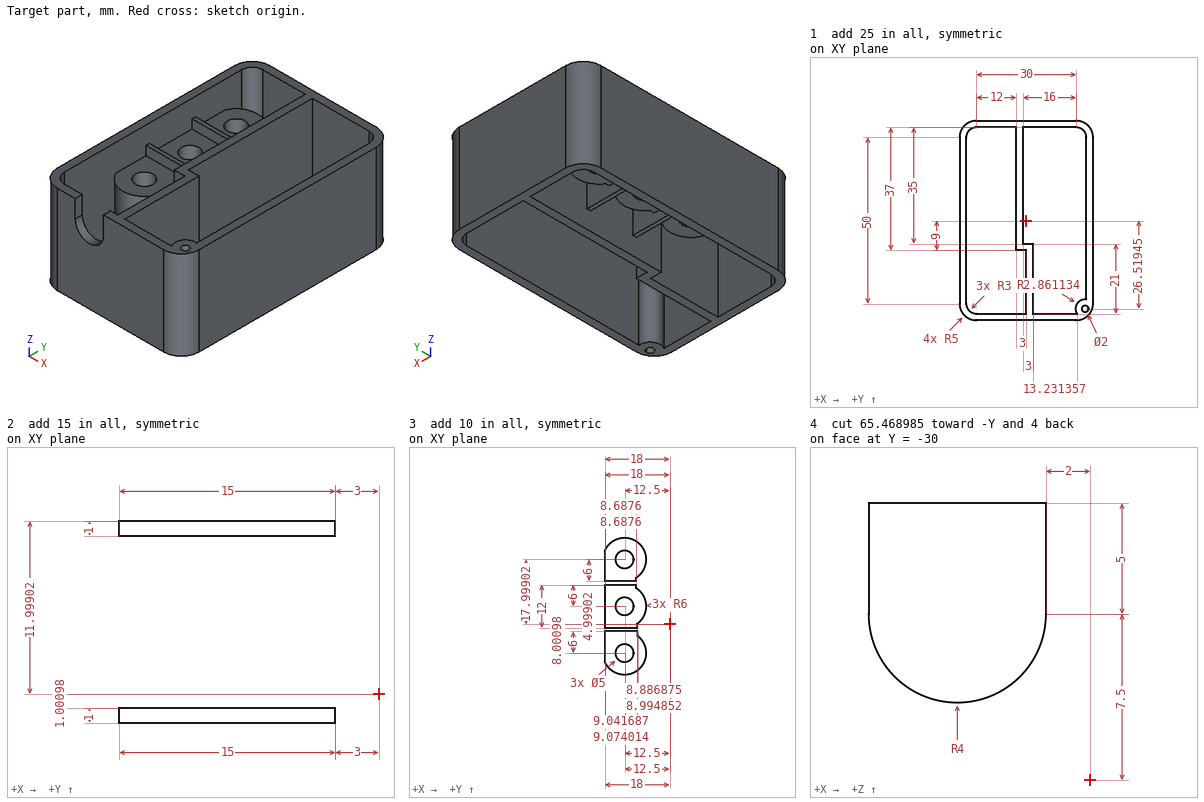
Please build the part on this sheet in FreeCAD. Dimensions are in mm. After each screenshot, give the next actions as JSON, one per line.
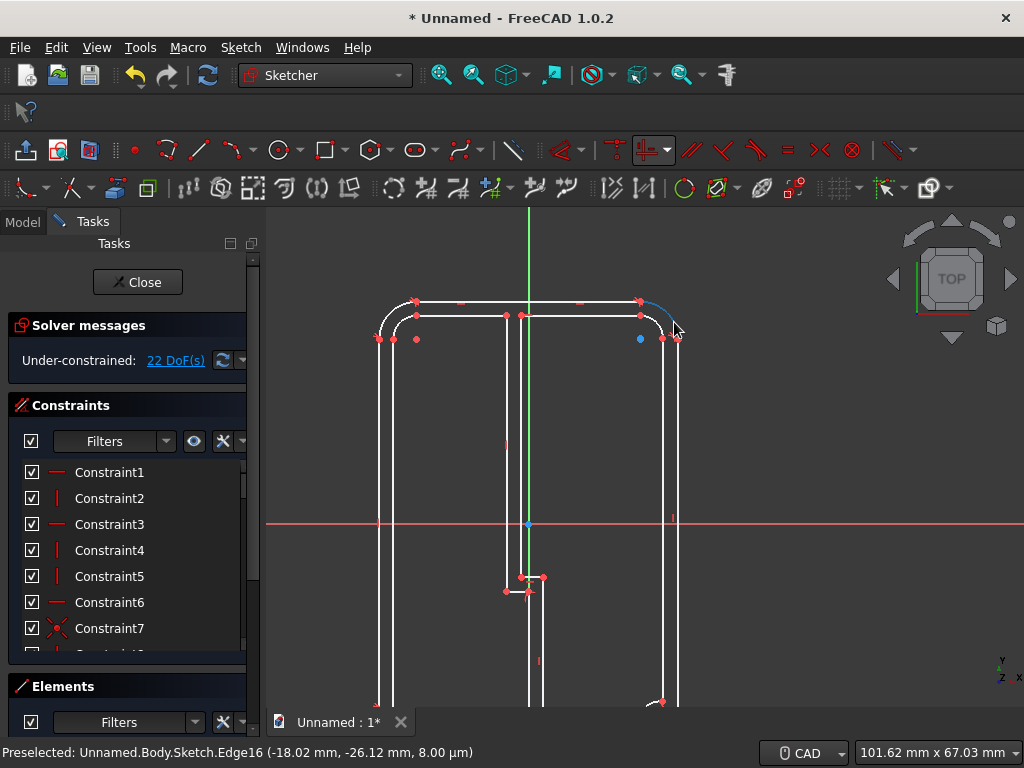
{"action": "left_click", "coordinate": [674, 322]}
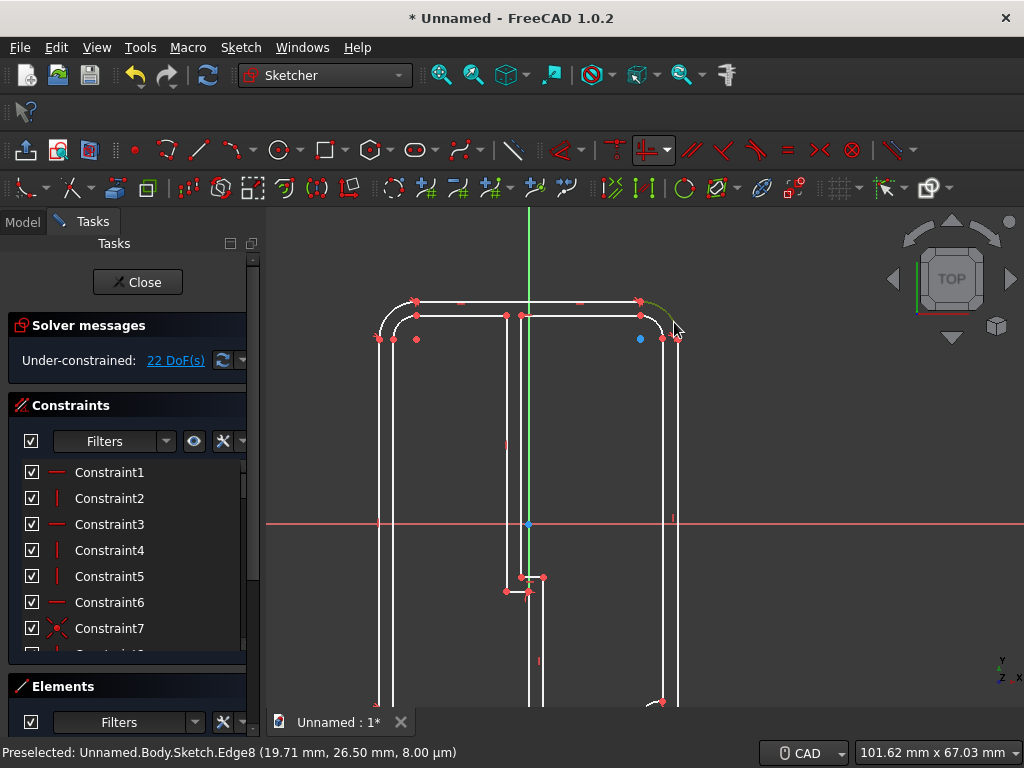
{"action": "scroll", "coordinate": [660, 328], "scroll_direction": "up", "scroll_amount": 2}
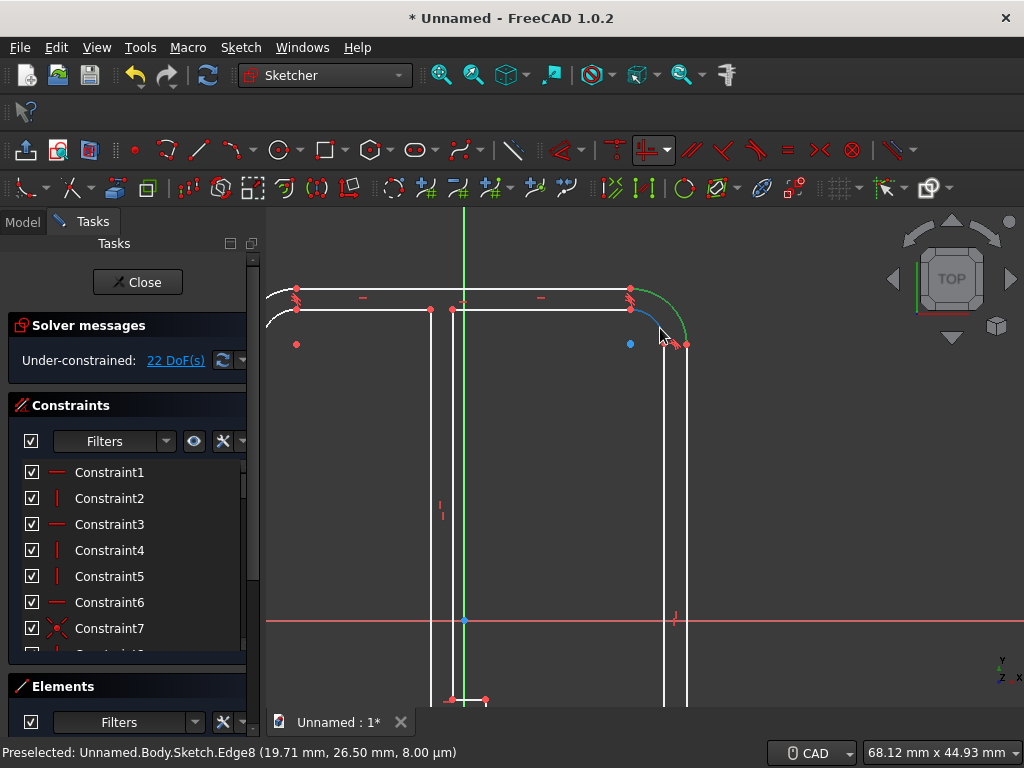
{"action": "left_click", "coordinate": [660, 328]}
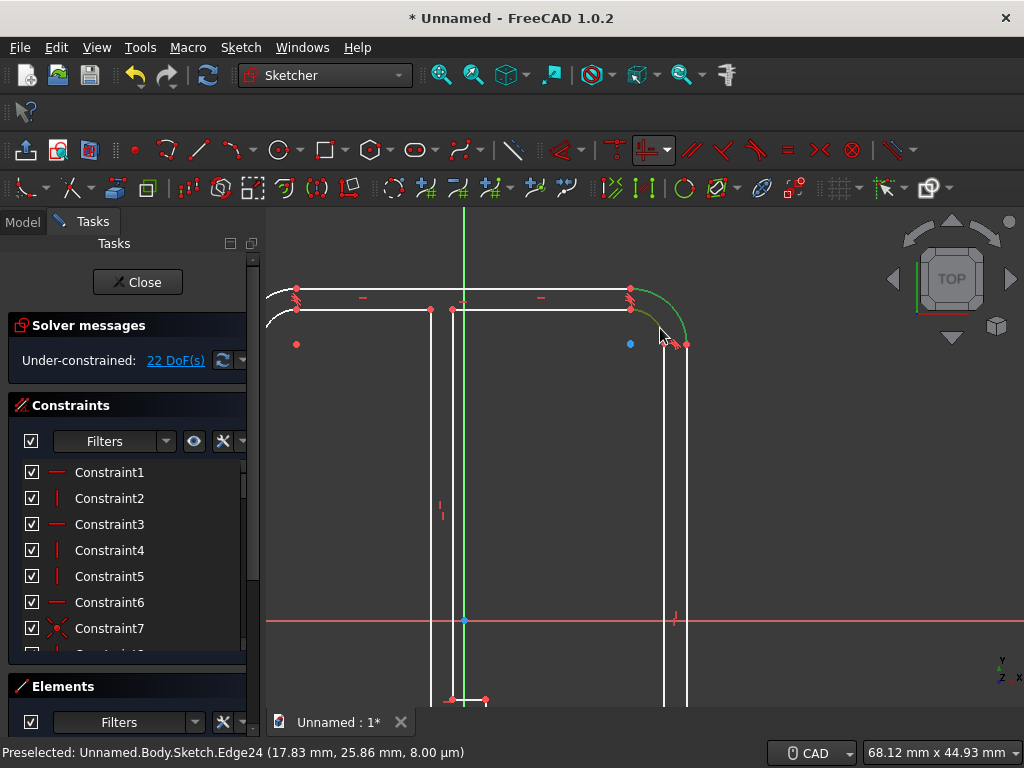
{"action": "left_click", "coordinate": [616, 150]}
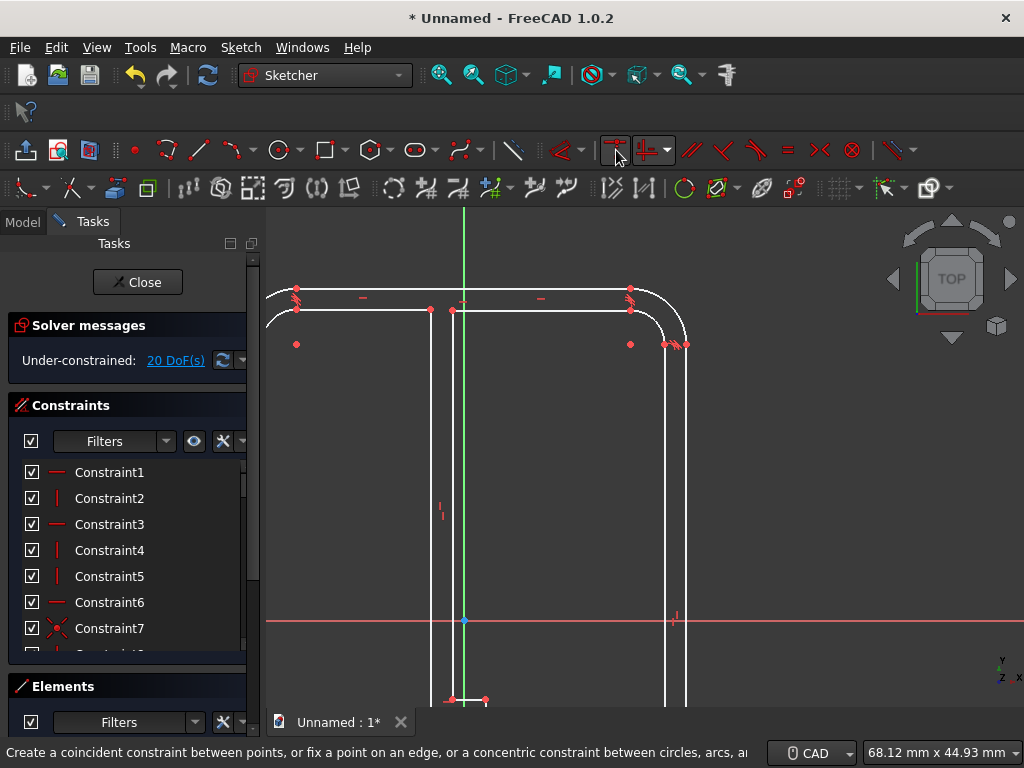
{"action": "scroll", "coordinate": [668, 324], "scroll_direction": "down", "scroll_amount": 4}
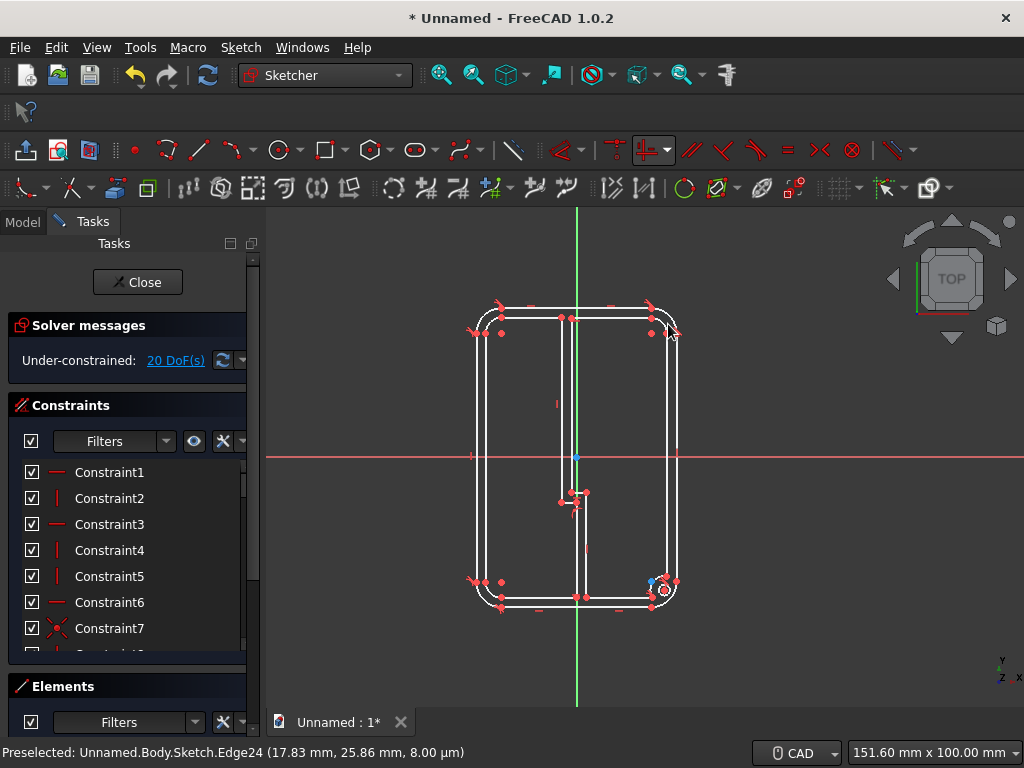
{"action": "scroll", "coordinate": [490, 311], "scroll_direction": "up", "scroll_amount": 2}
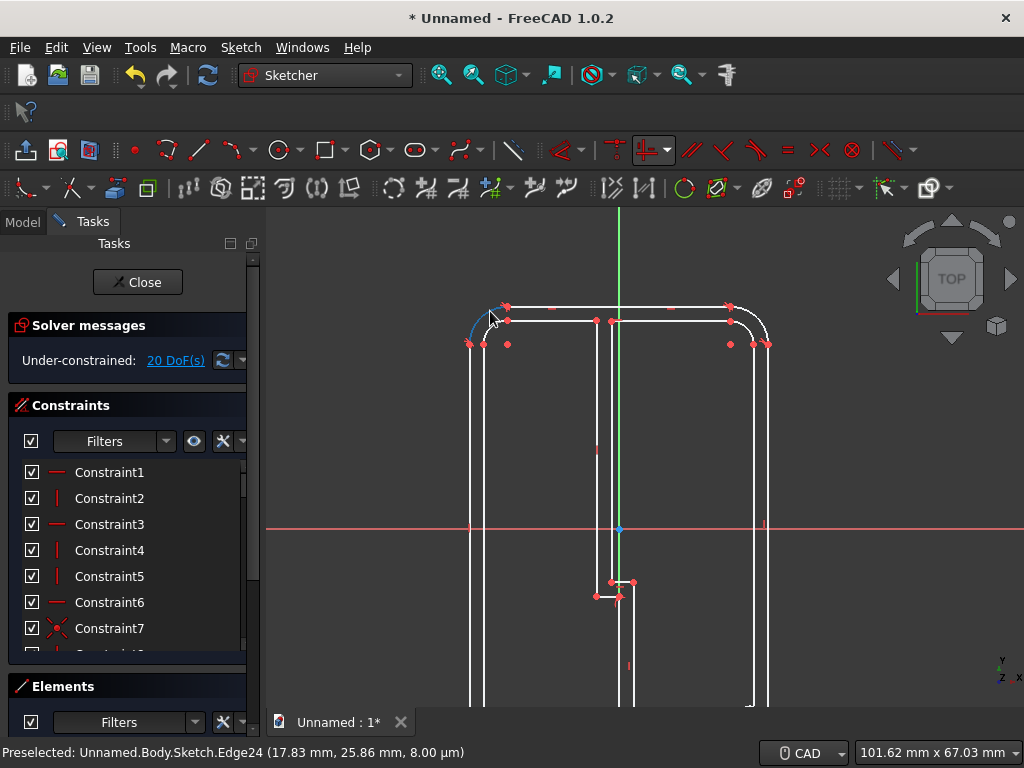
{"action": "left_click", "coordinate": [490, 311]}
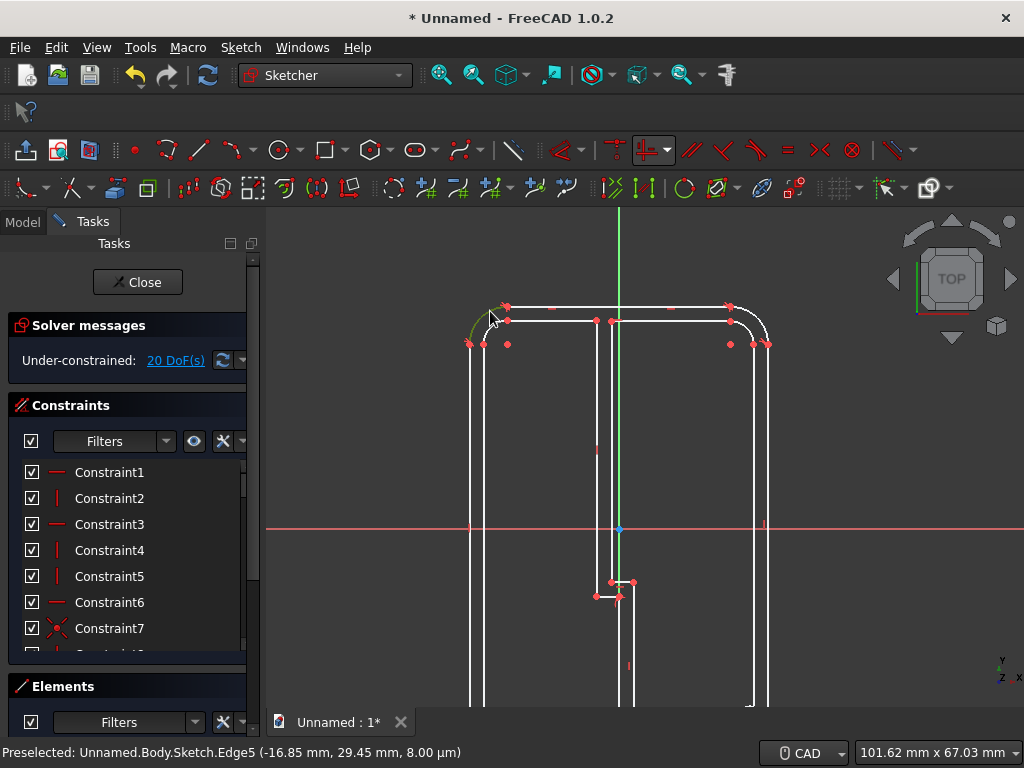
{"action": "scroll", "coordinate": [490, 310], "scroll_direction": "down", "scroll_amount": 2}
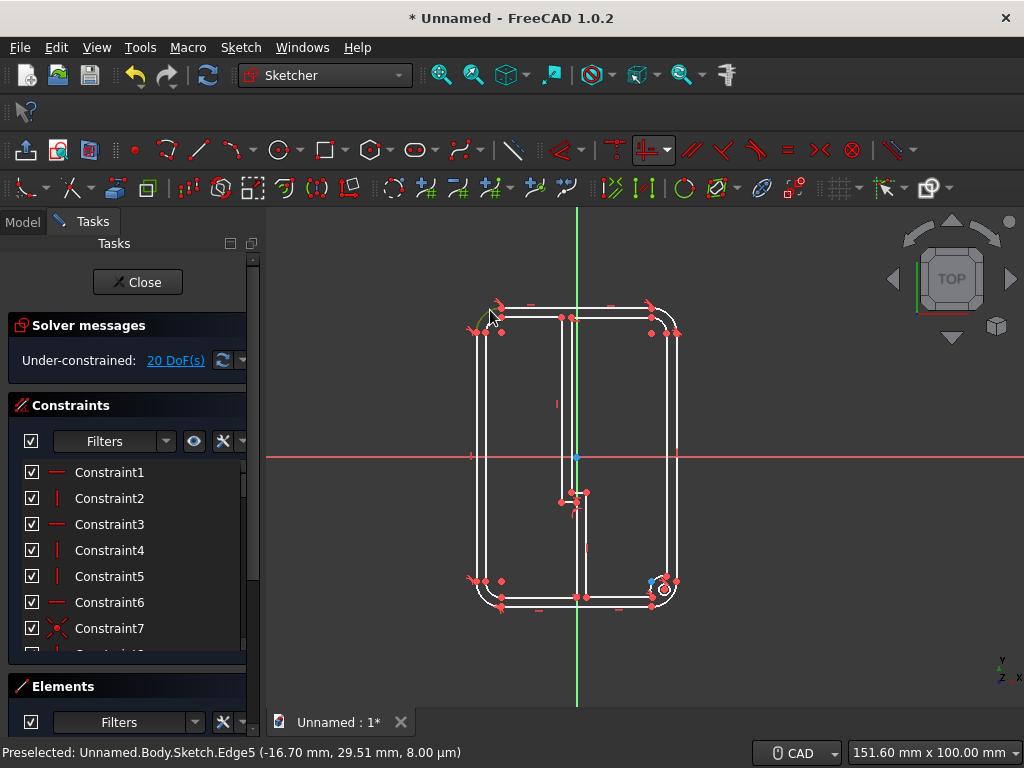
{"action": "scroll", "coordinate": [479, 593], "scroll_direction": "up", "scroll_amount": 2}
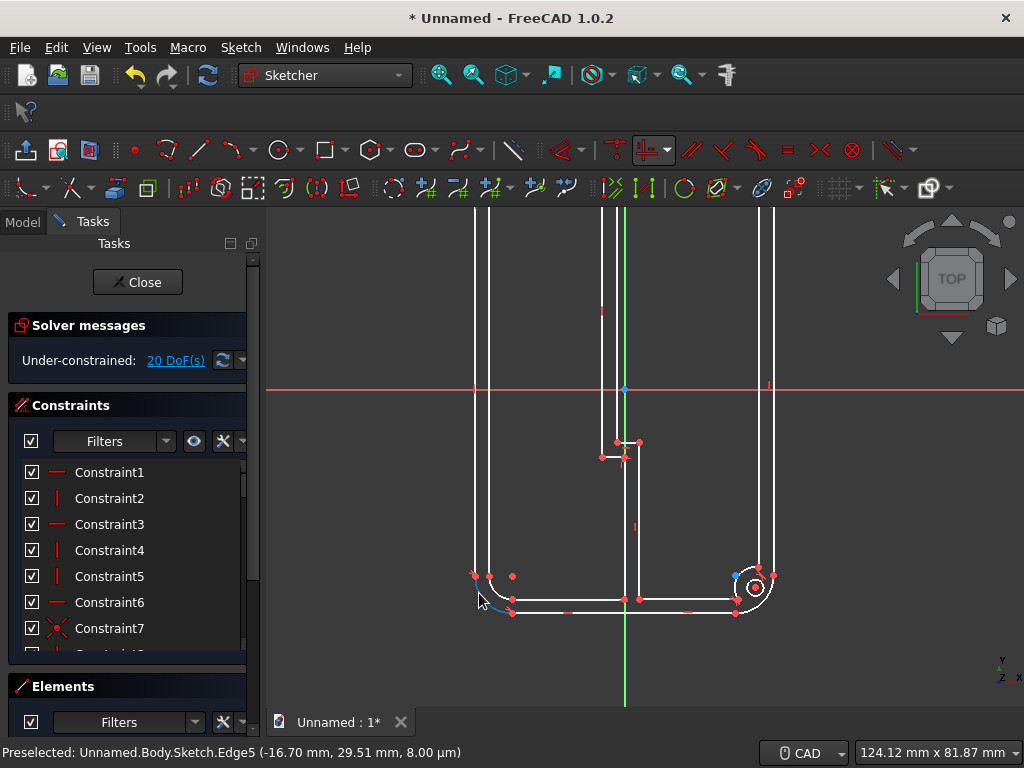
{"action": "left_click", "coordinate": [479, 593]}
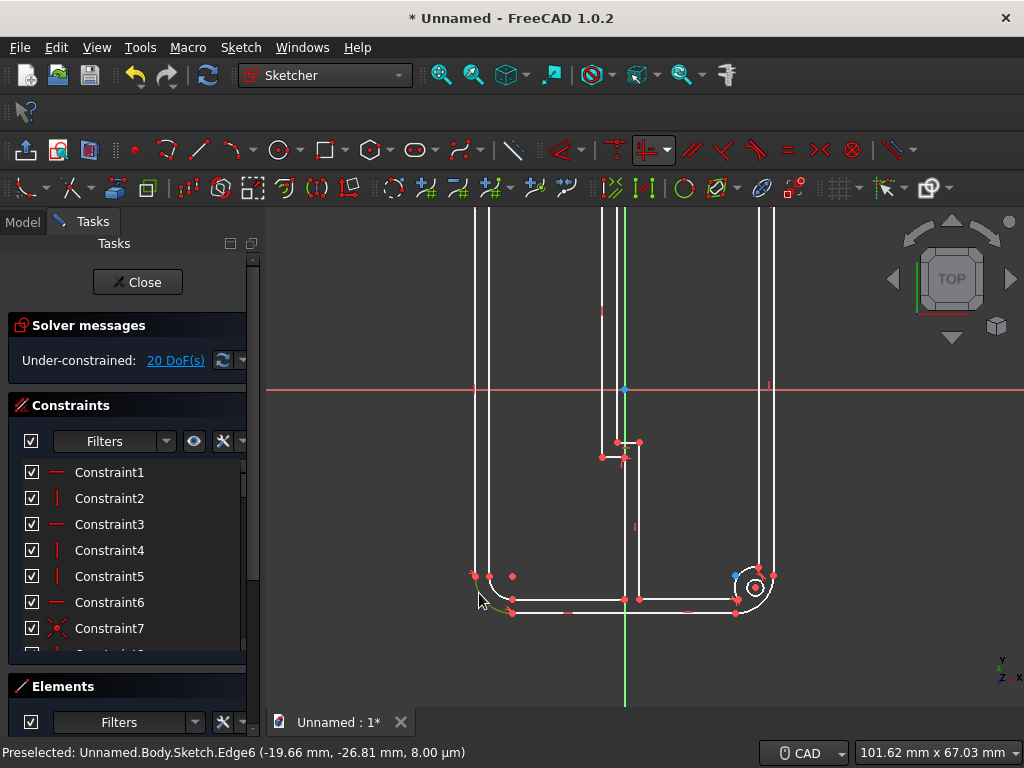
{"action": "left_click", "coordinate": [753, 609]}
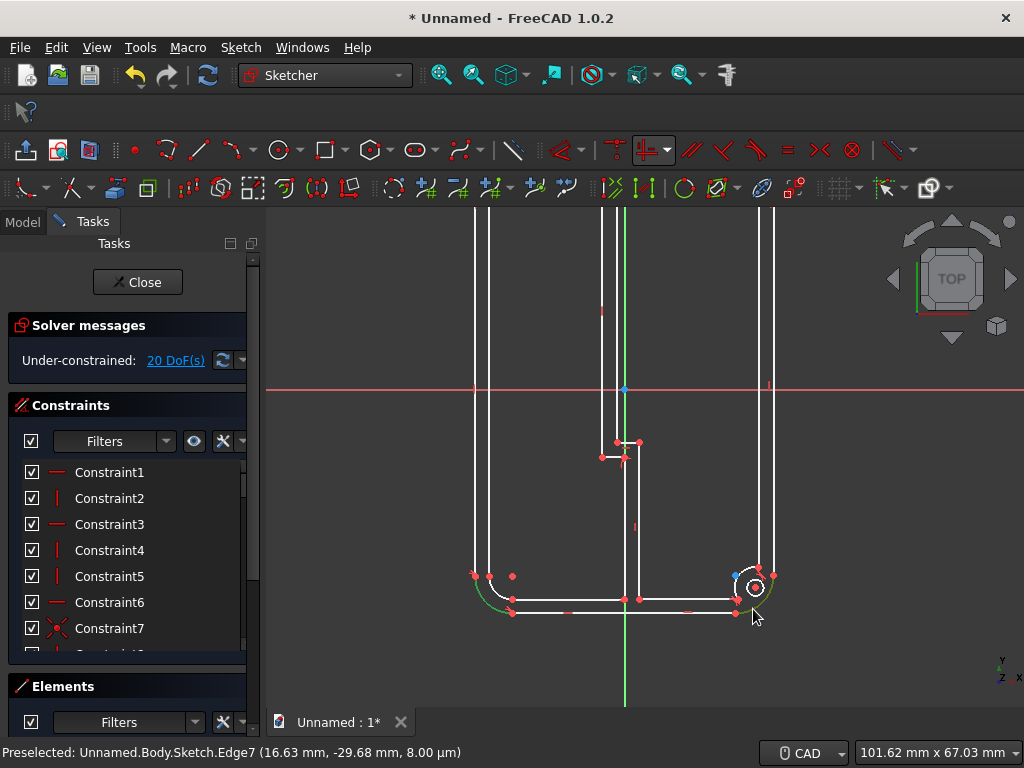
{"action": "scroll", "coordinate": [479, 594], "scroll_direction": "down", "scroll_amount": 2}